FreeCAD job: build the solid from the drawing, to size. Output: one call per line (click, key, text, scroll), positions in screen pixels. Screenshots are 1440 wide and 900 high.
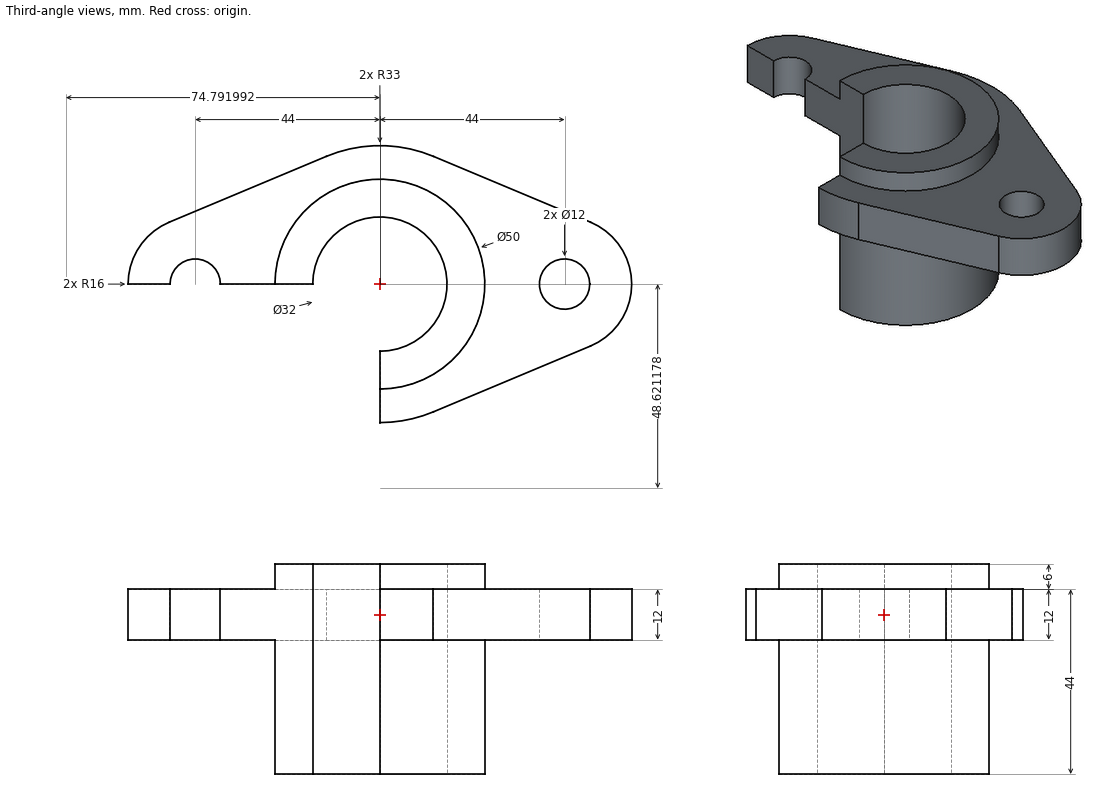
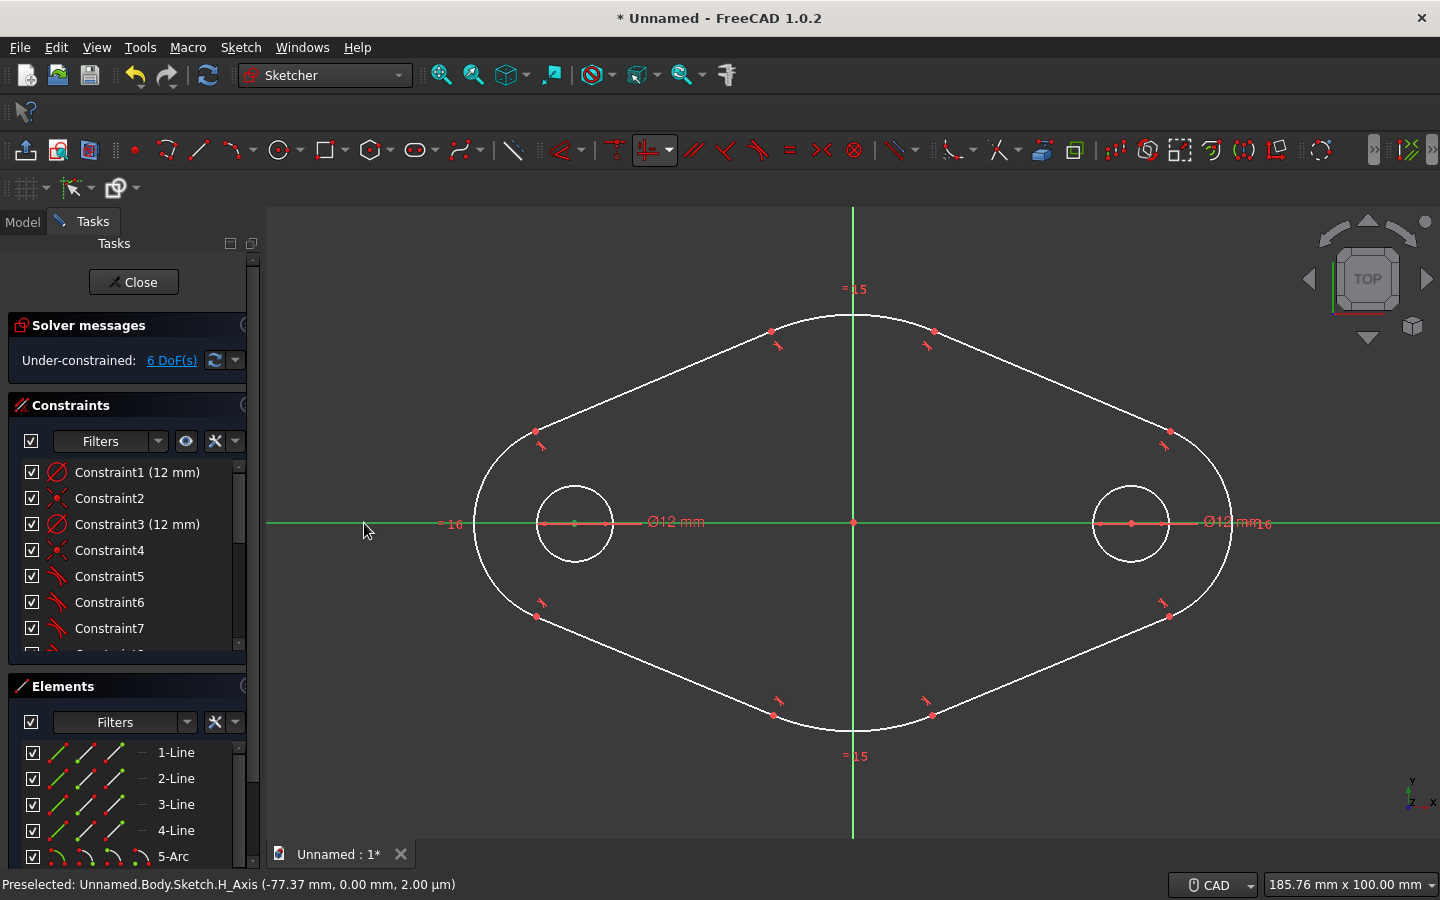
key(c)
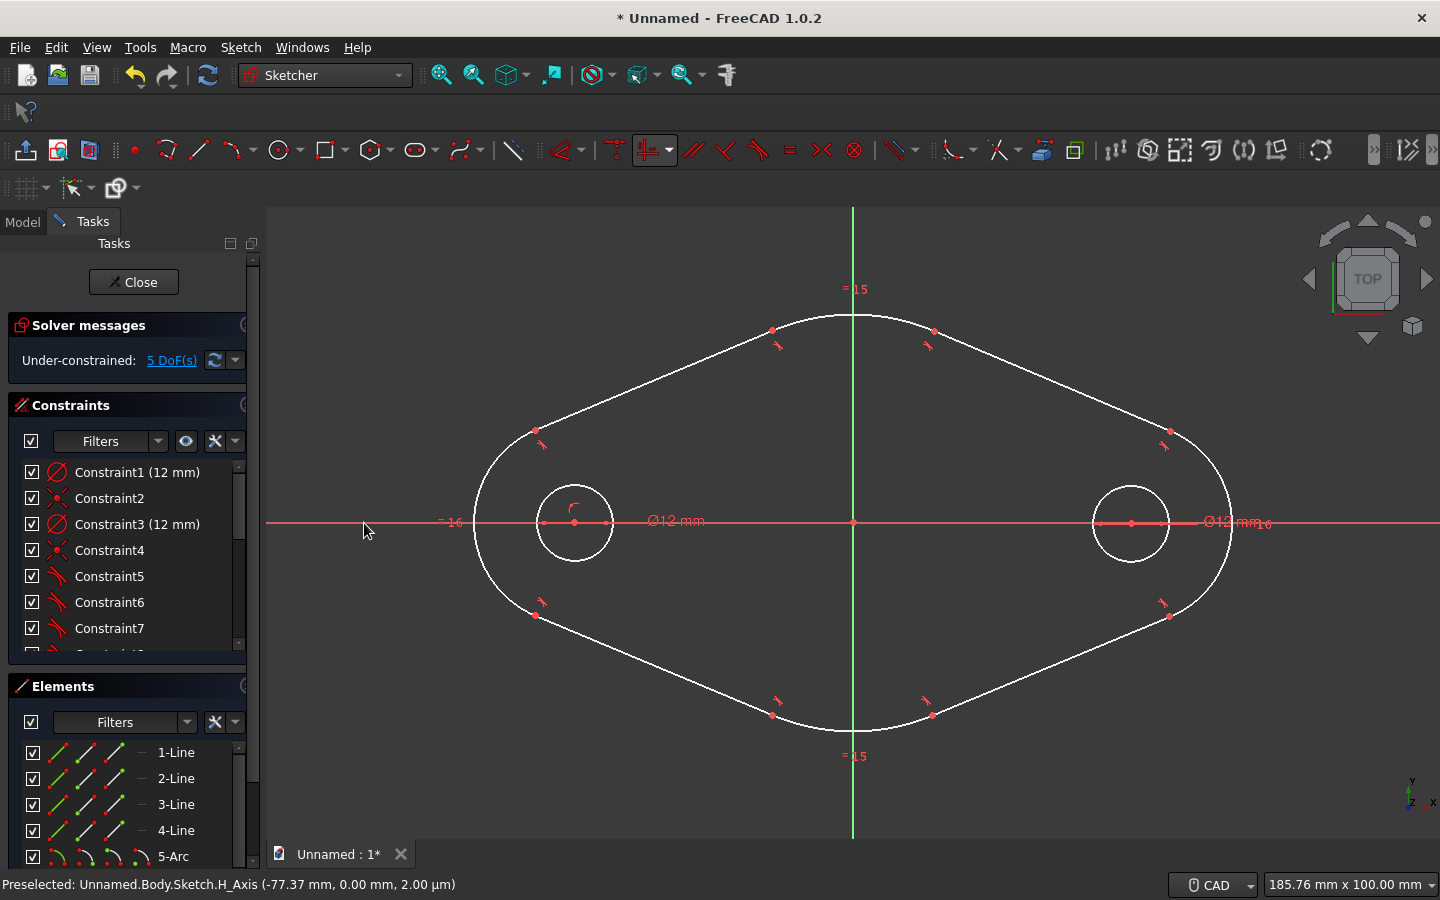
click(1131, 524)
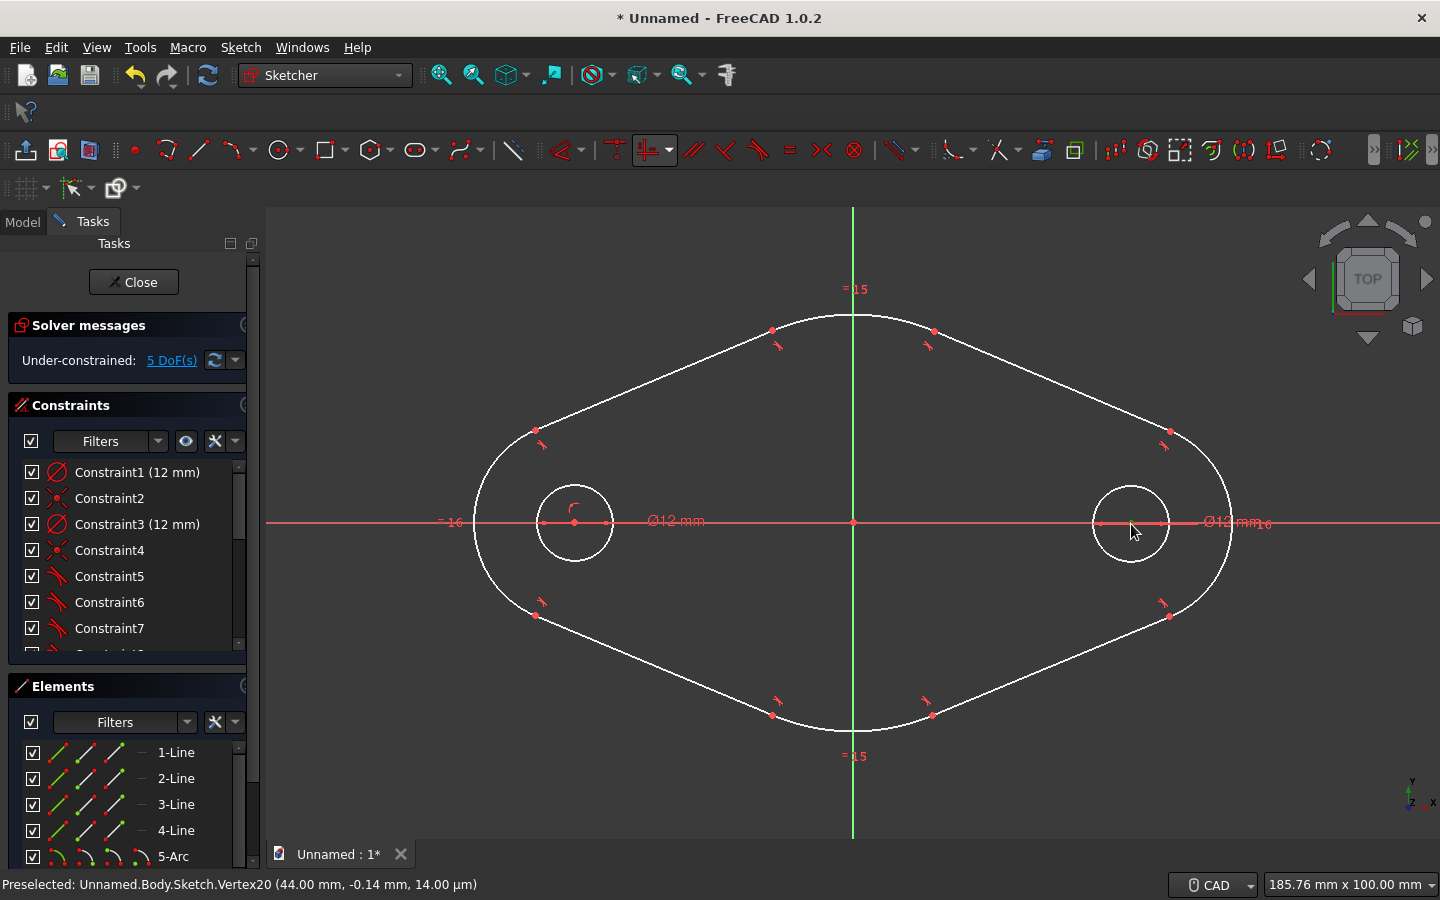
click(364, 523)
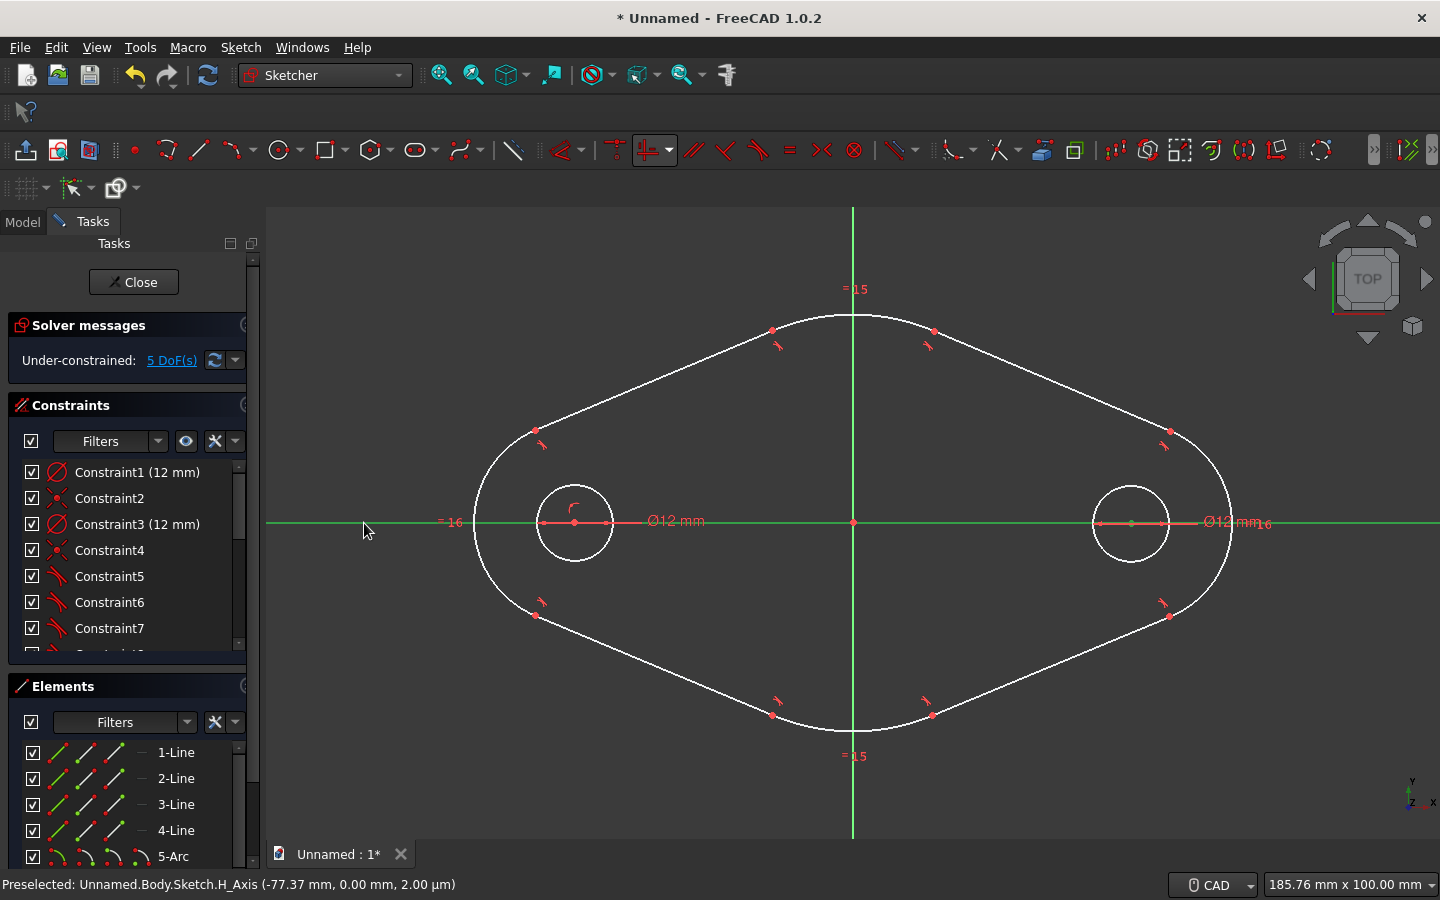
click(616, 150)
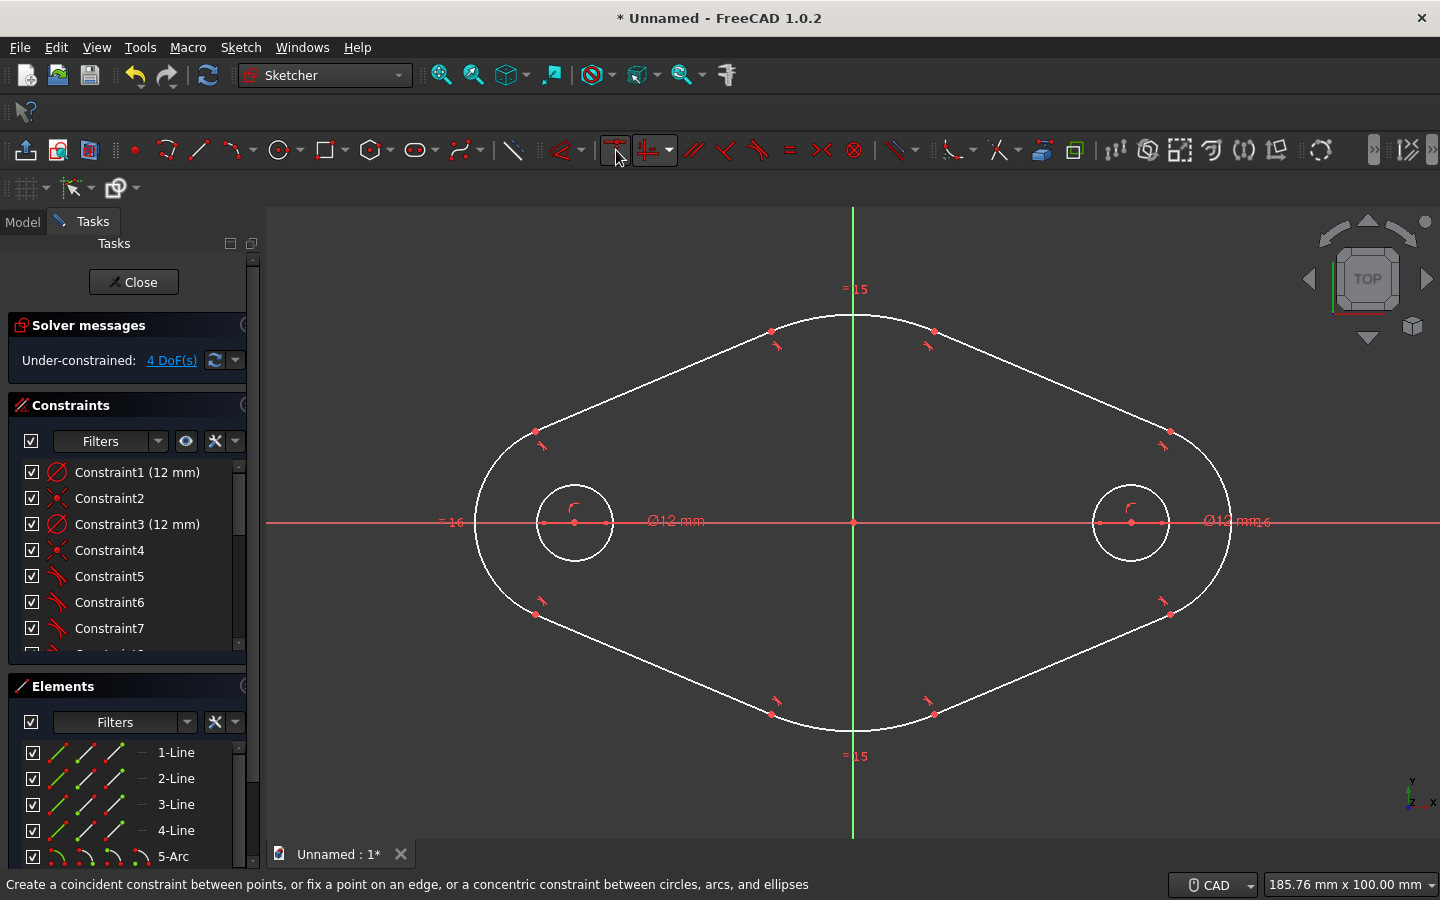
click(560, 150)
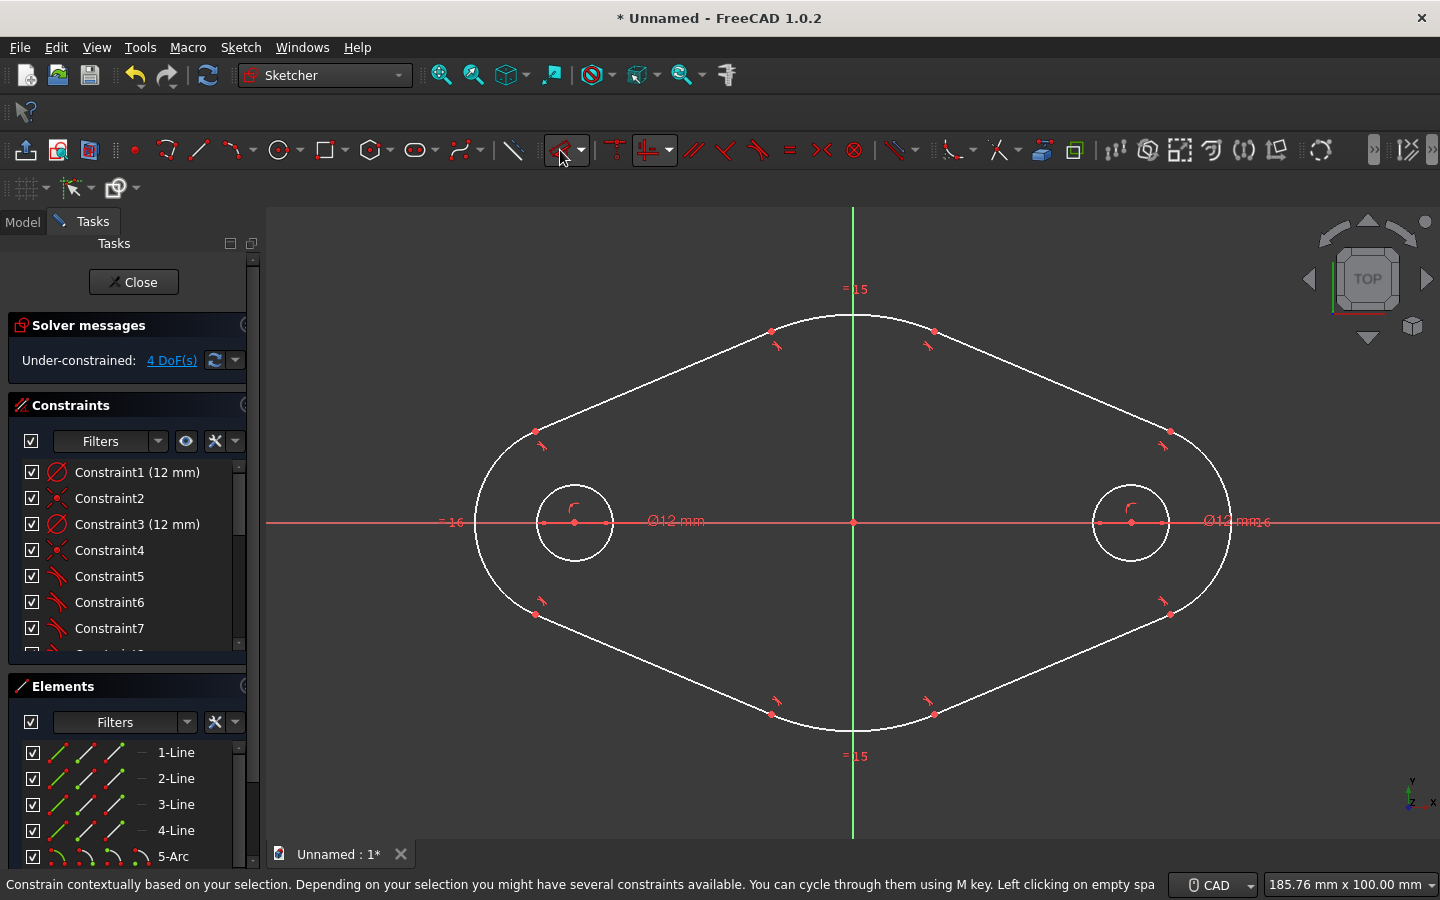
click(886, 317)
click(891, 285)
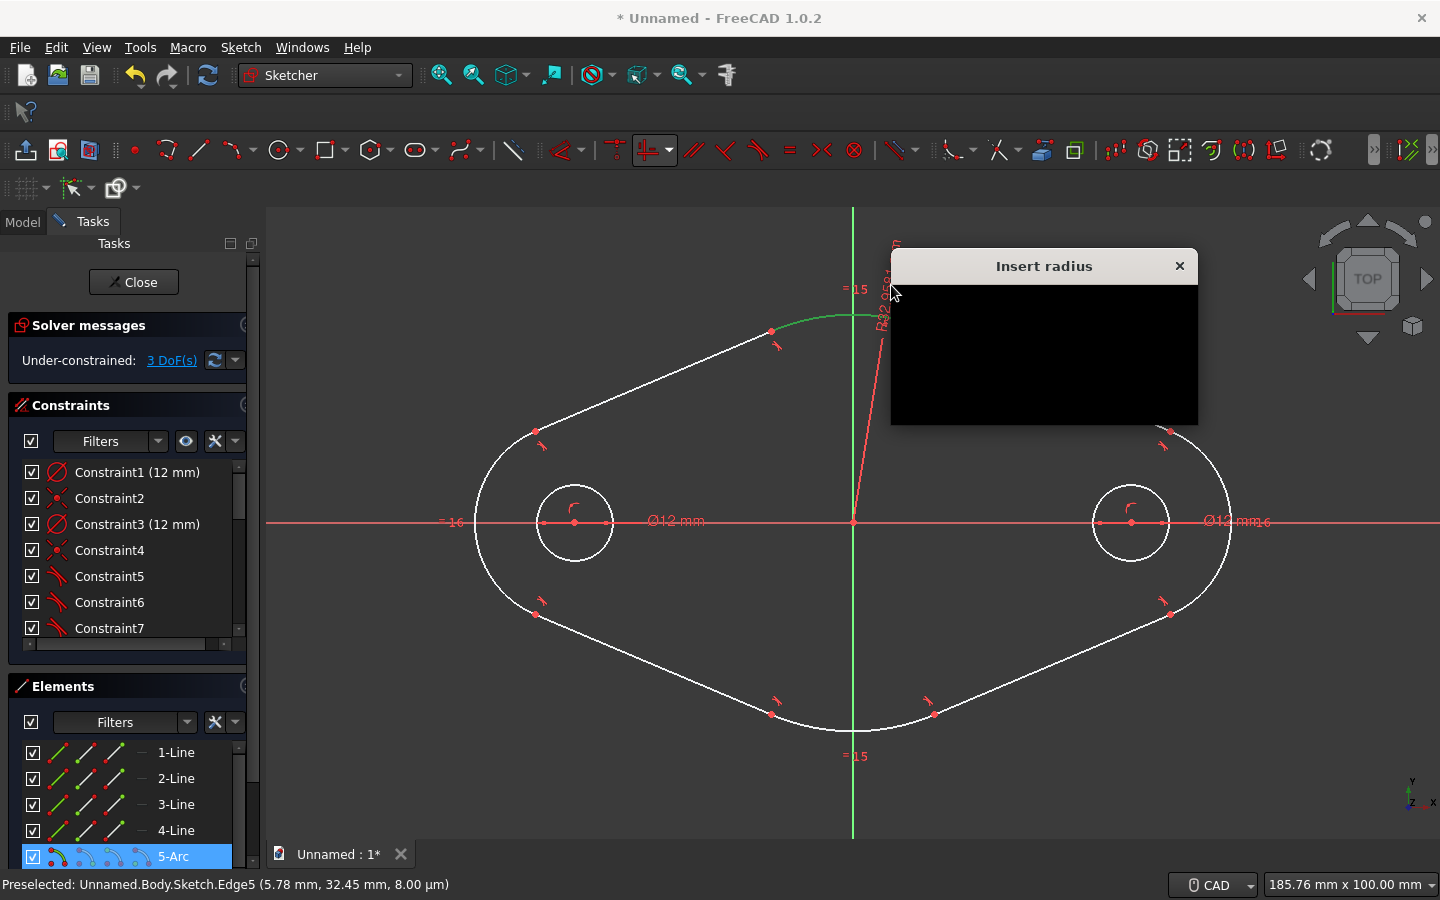
text(33)
key(Return)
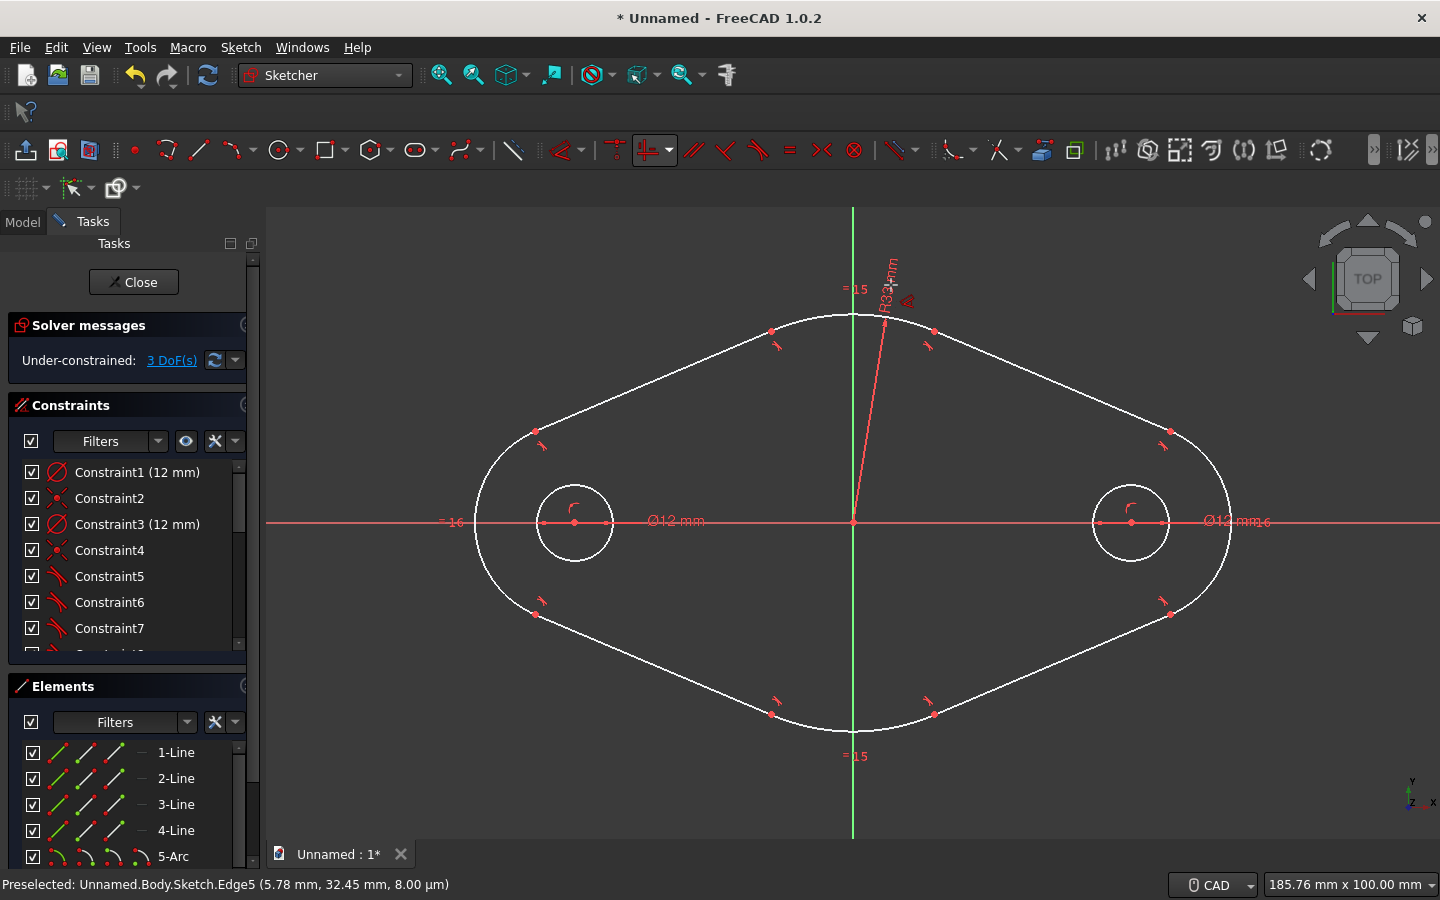
click(486, 478)
click(457, 464)